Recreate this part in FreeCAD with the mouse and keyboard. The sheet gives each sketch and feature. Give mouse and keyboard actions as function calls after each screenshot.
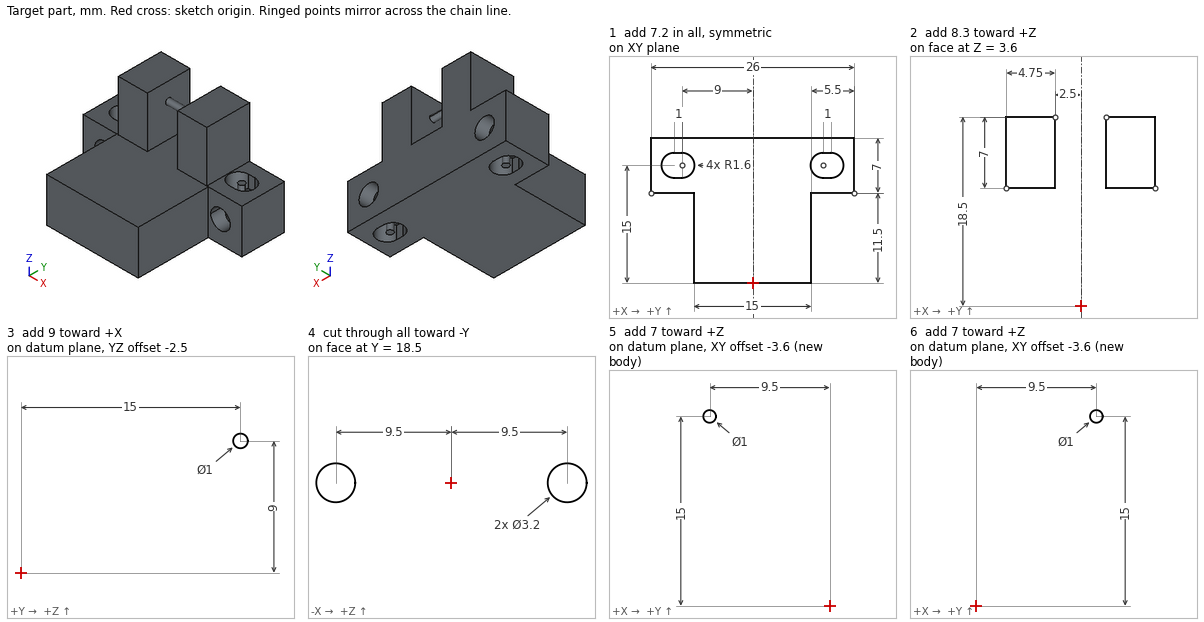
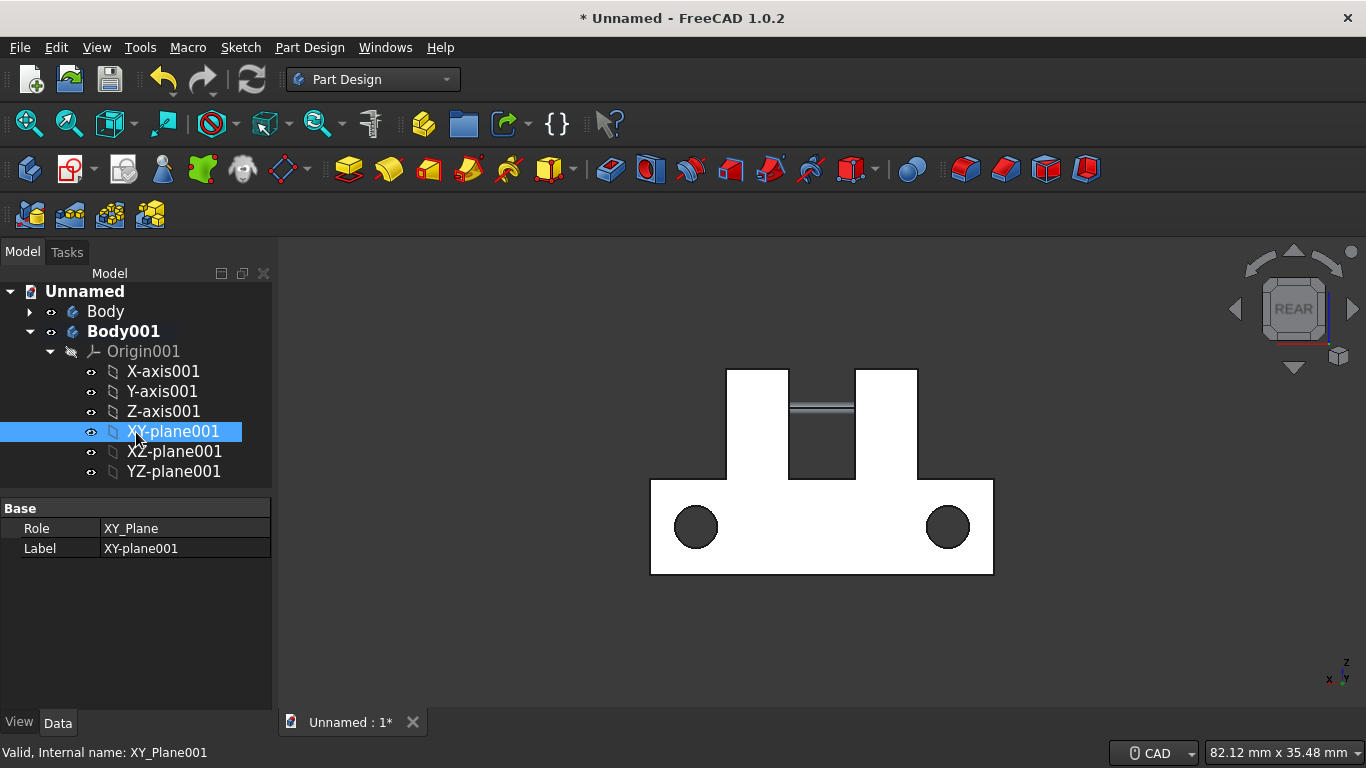
click(284, 170)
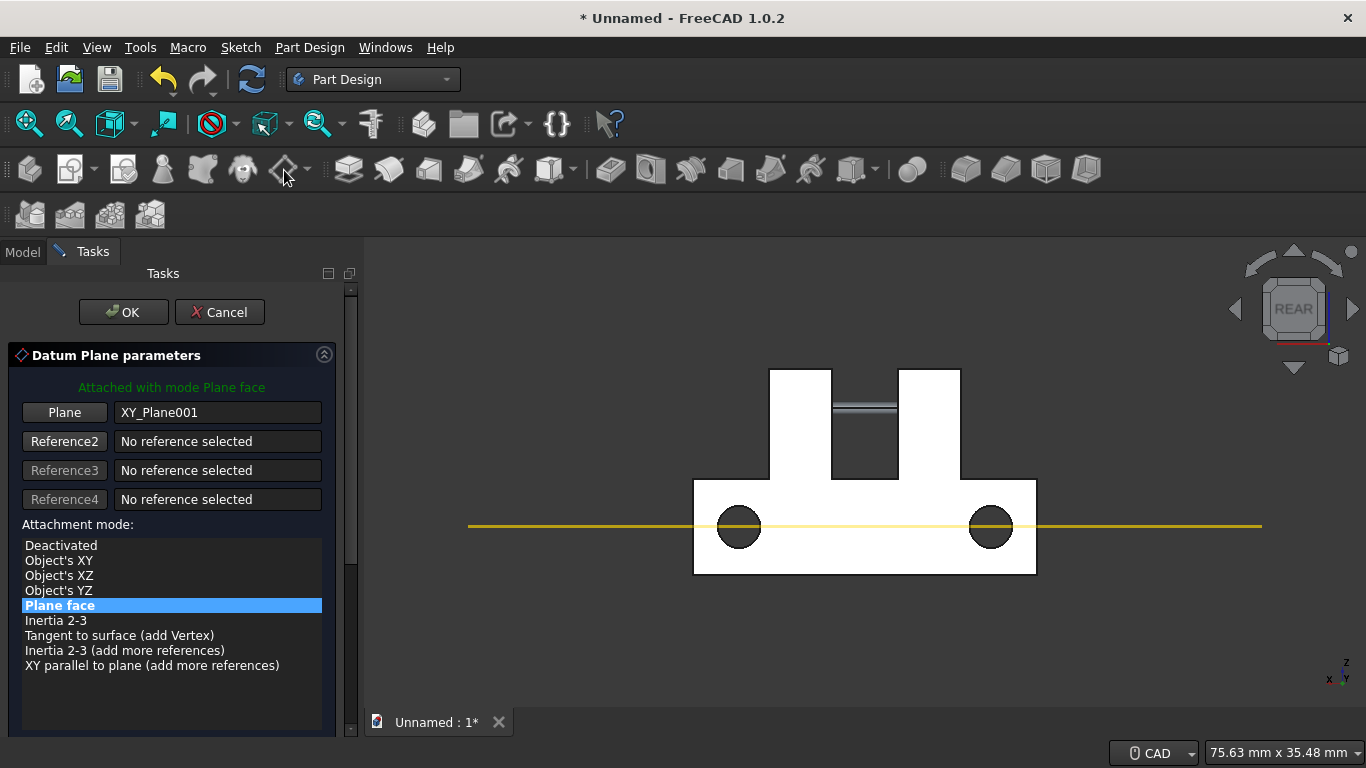
scroll(351, 510, down, 3)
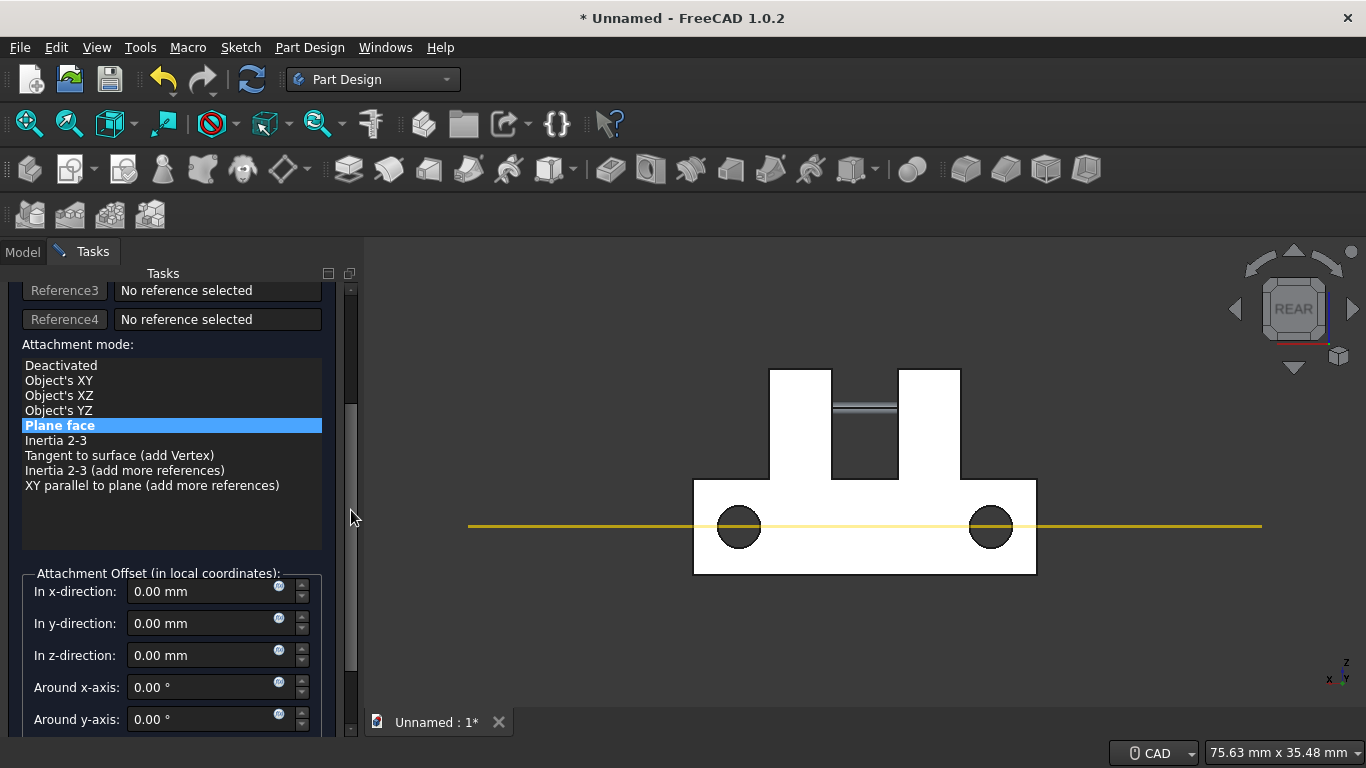
triple_click(210, 655)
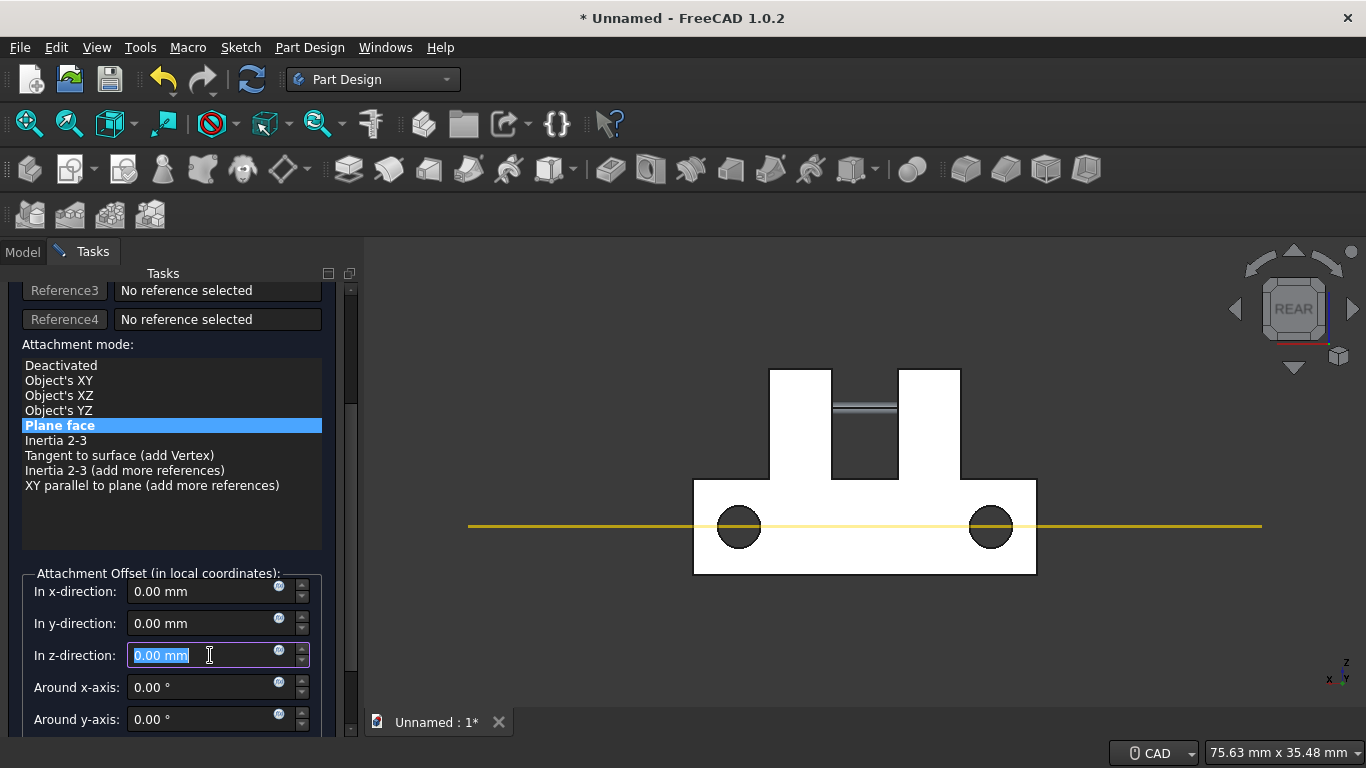
text(-3.6)
key(Tab)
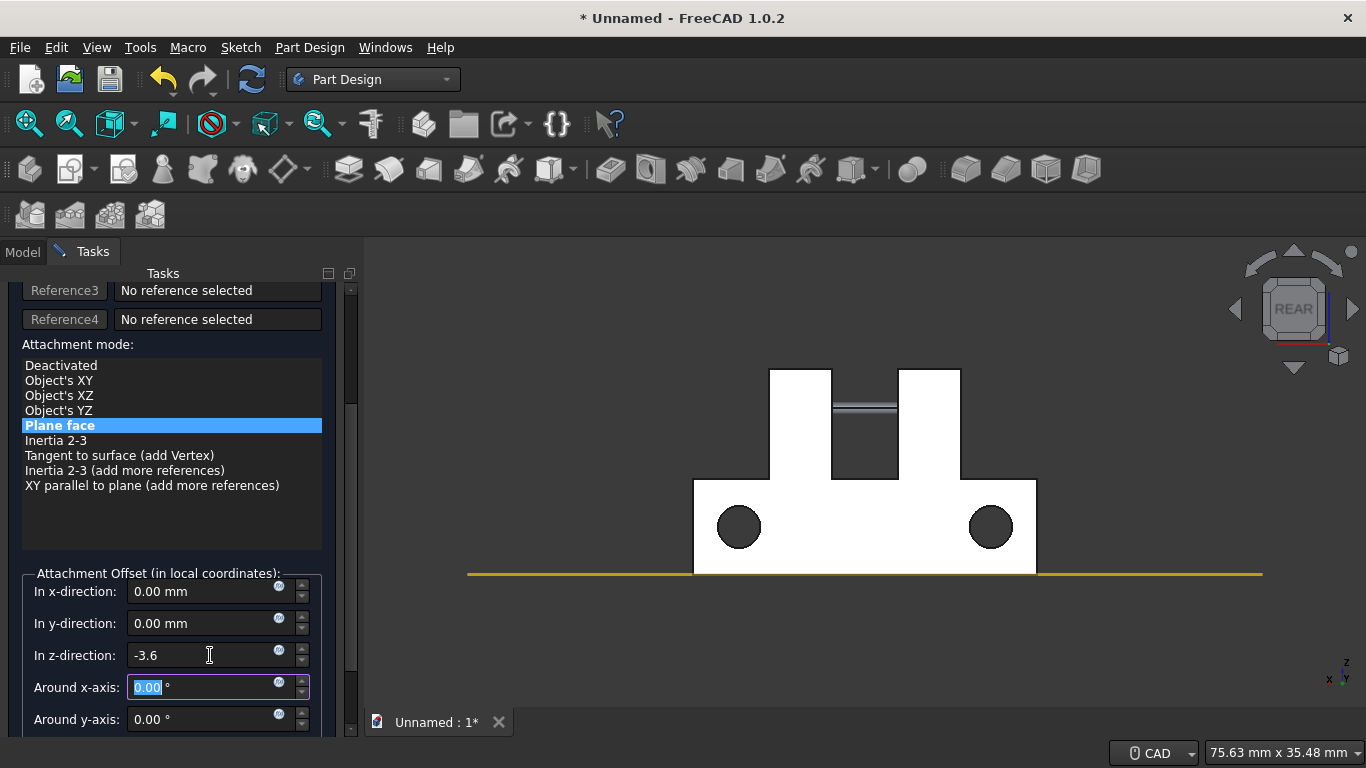
scroll(351, 510, up, 4)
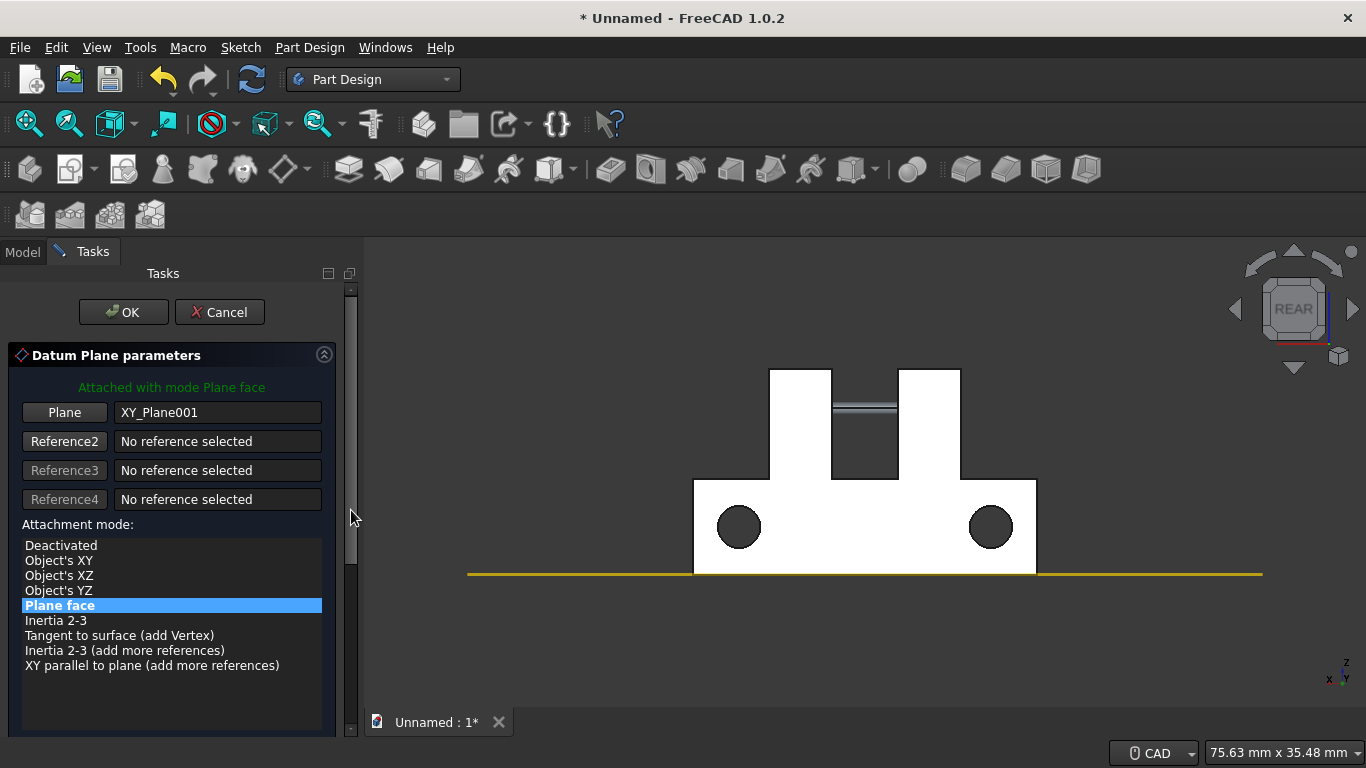
click(124, 312)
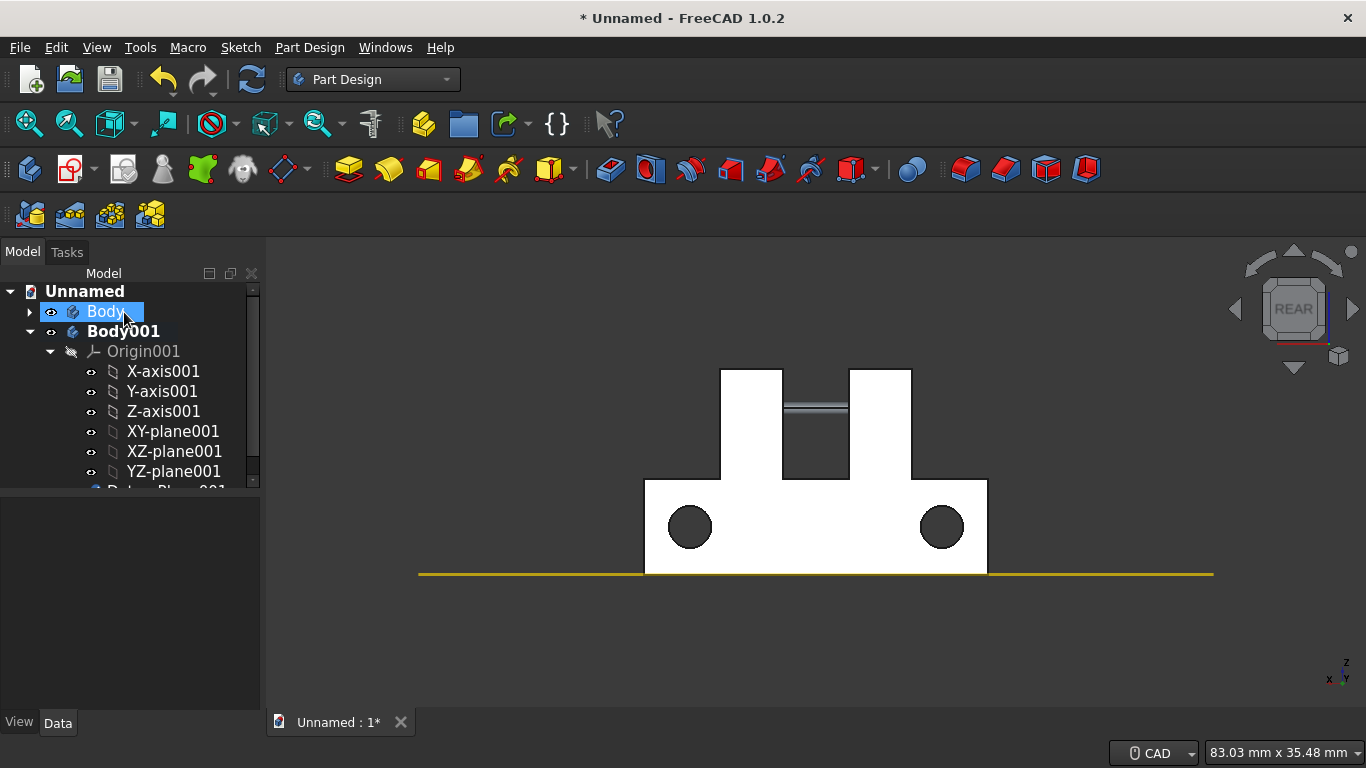
scroll(100, 387, down, 3)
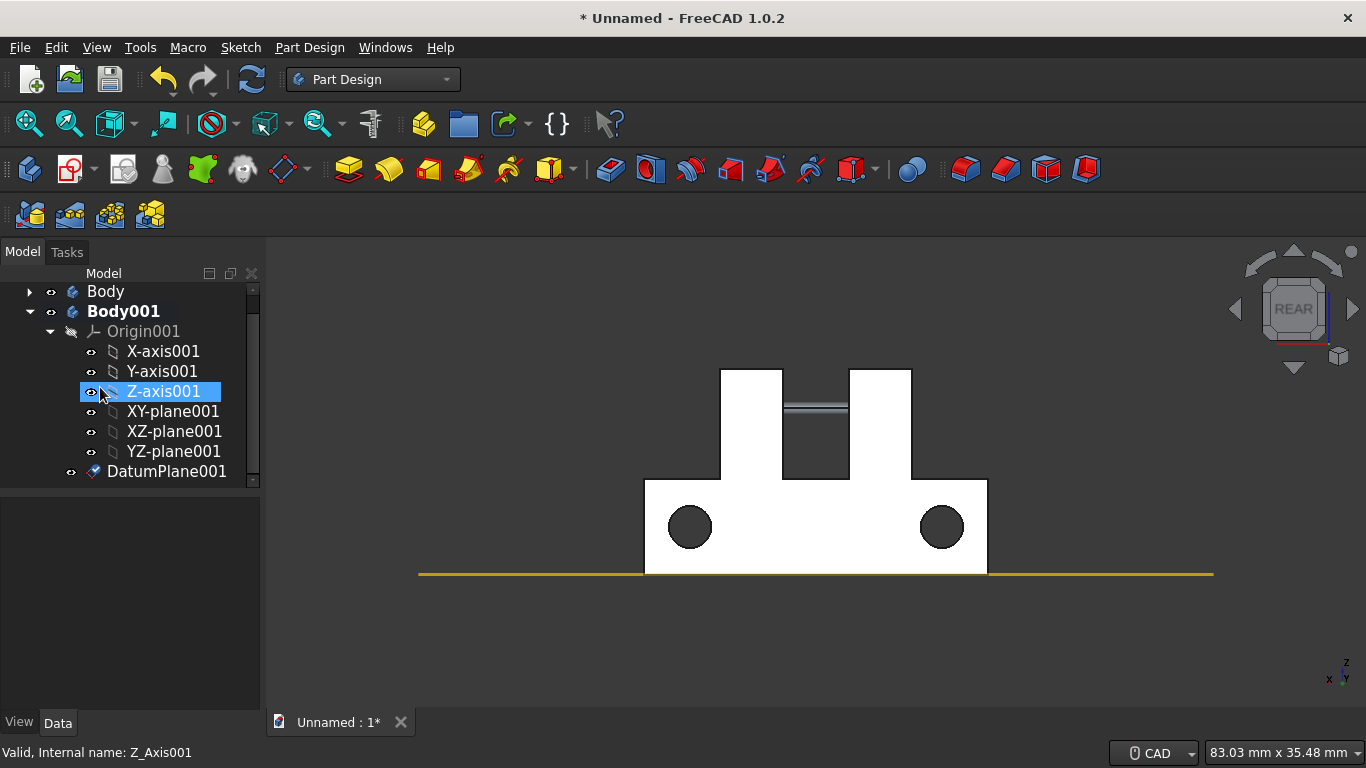
click(116, 472)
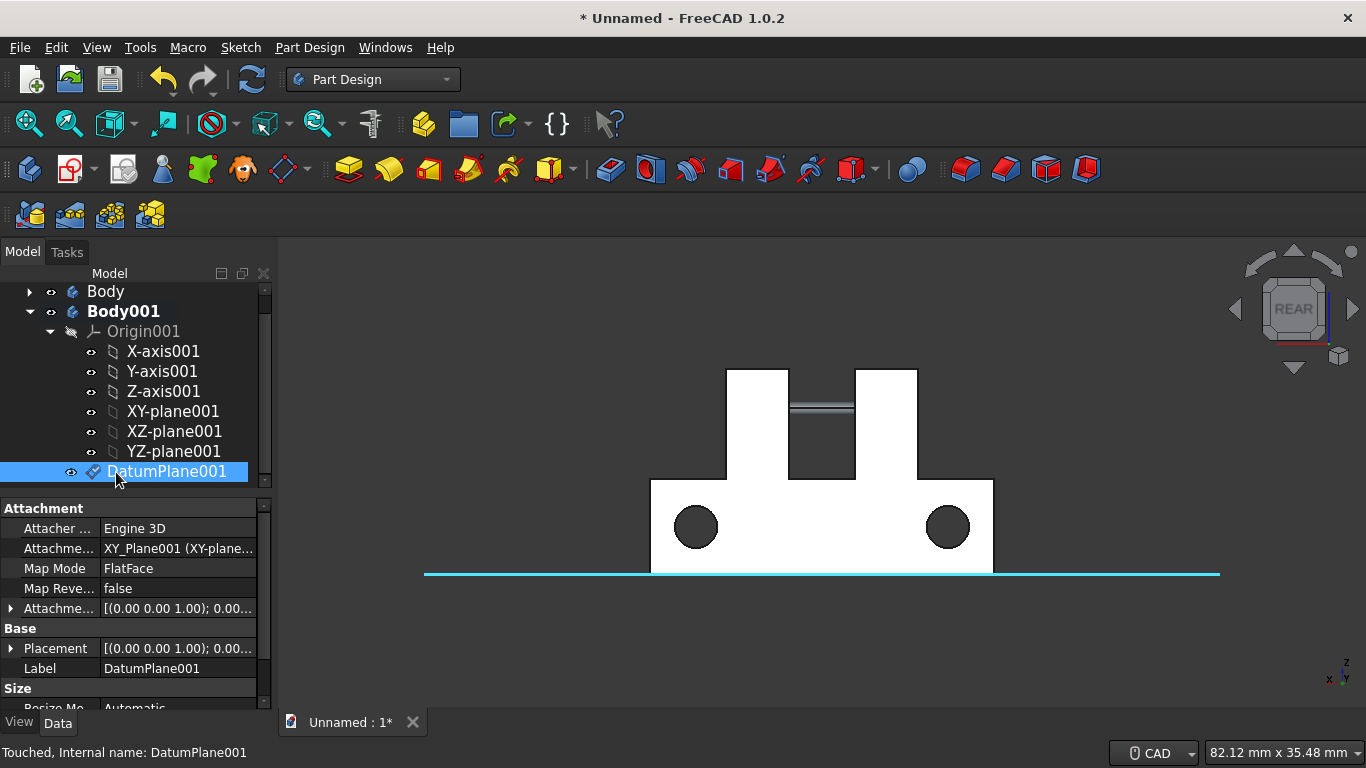
click(70, 170)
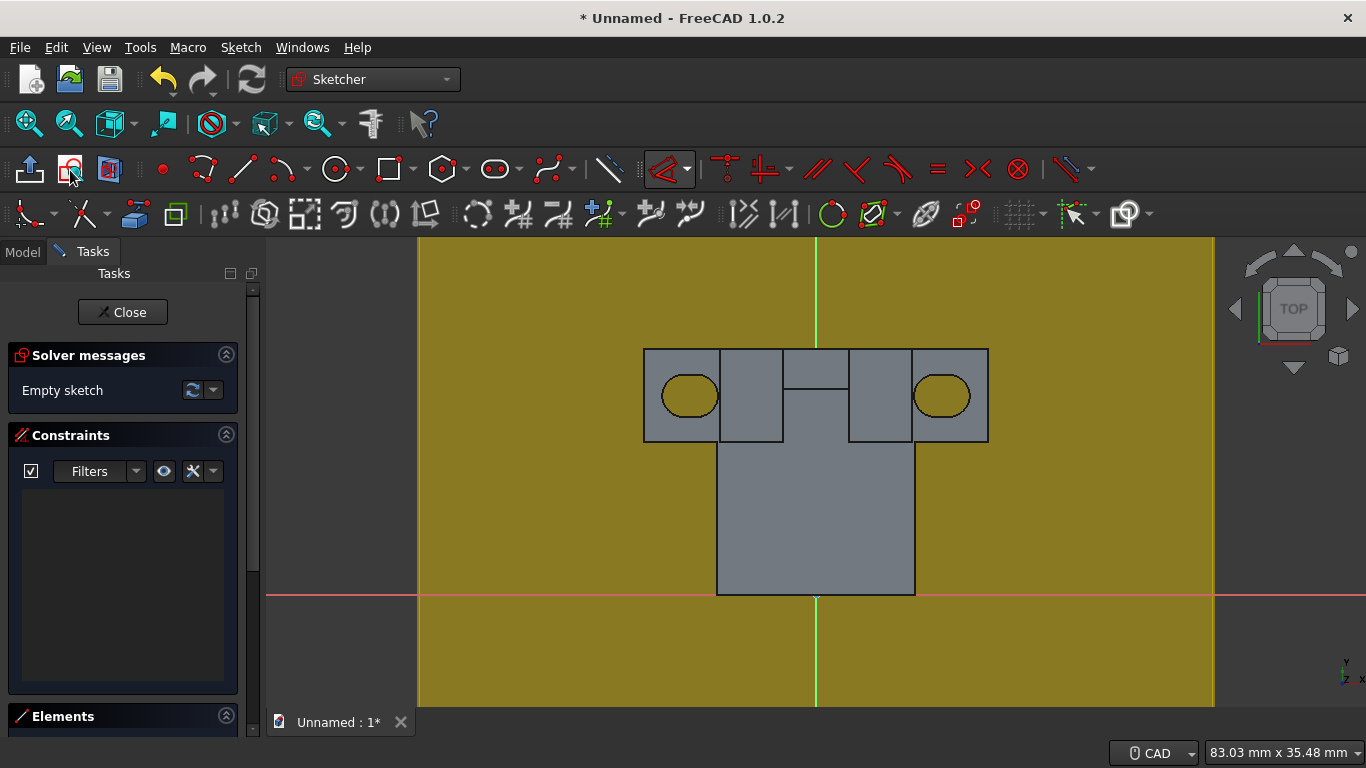
scroll(687, 392, up, 15)